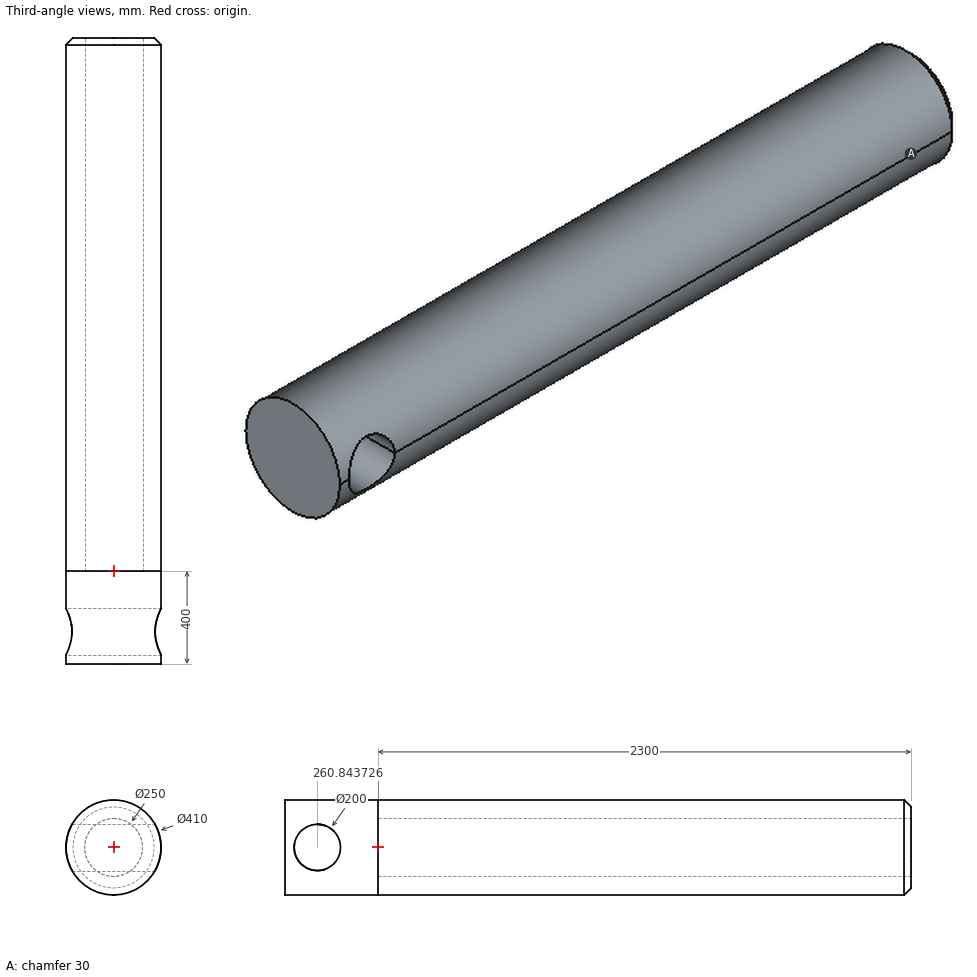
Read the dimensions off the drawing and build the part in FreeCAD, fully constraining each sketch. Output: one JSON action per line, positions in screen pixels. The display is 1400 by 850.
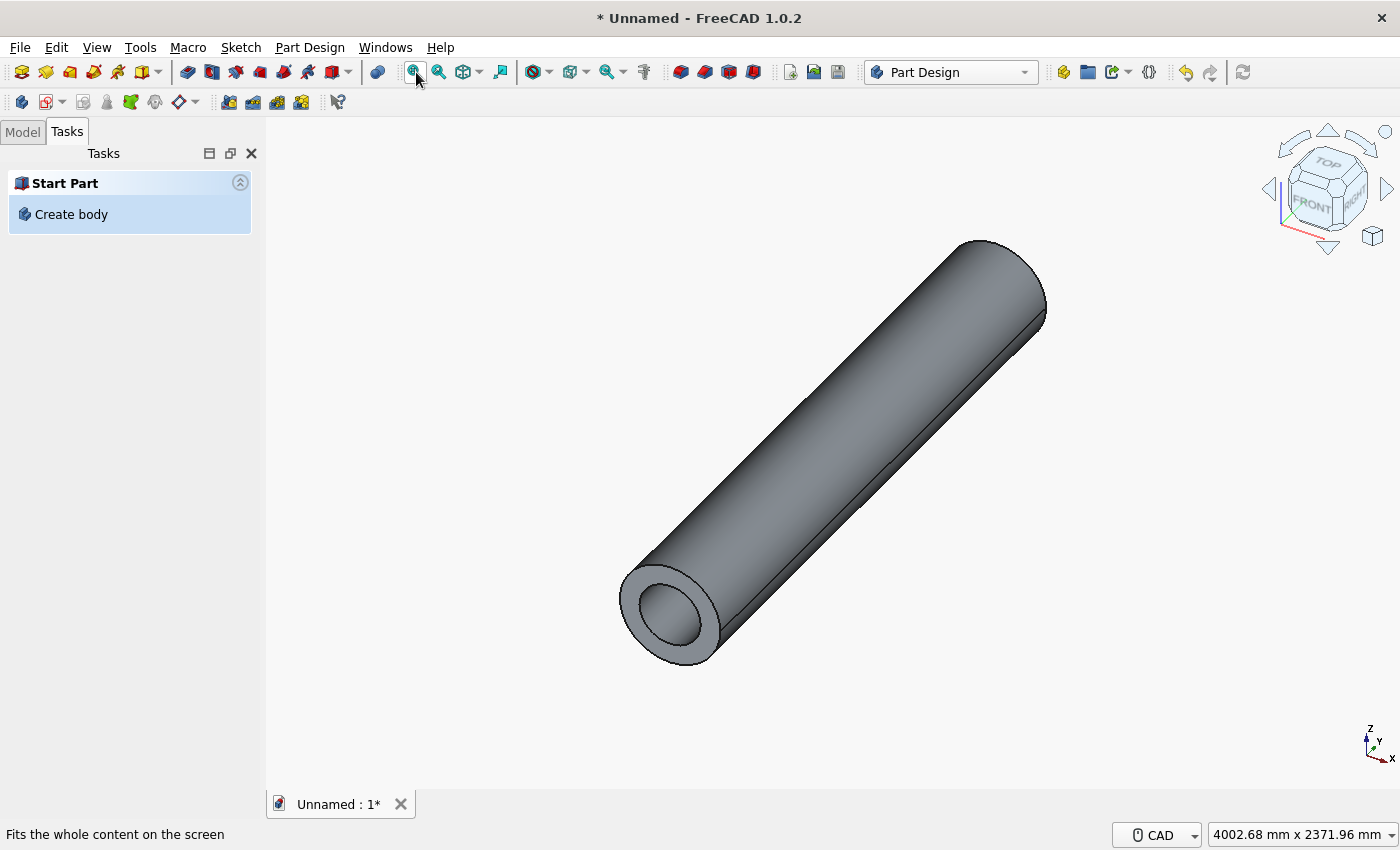
{"action": "left_click", "coordinate": [23, 131]}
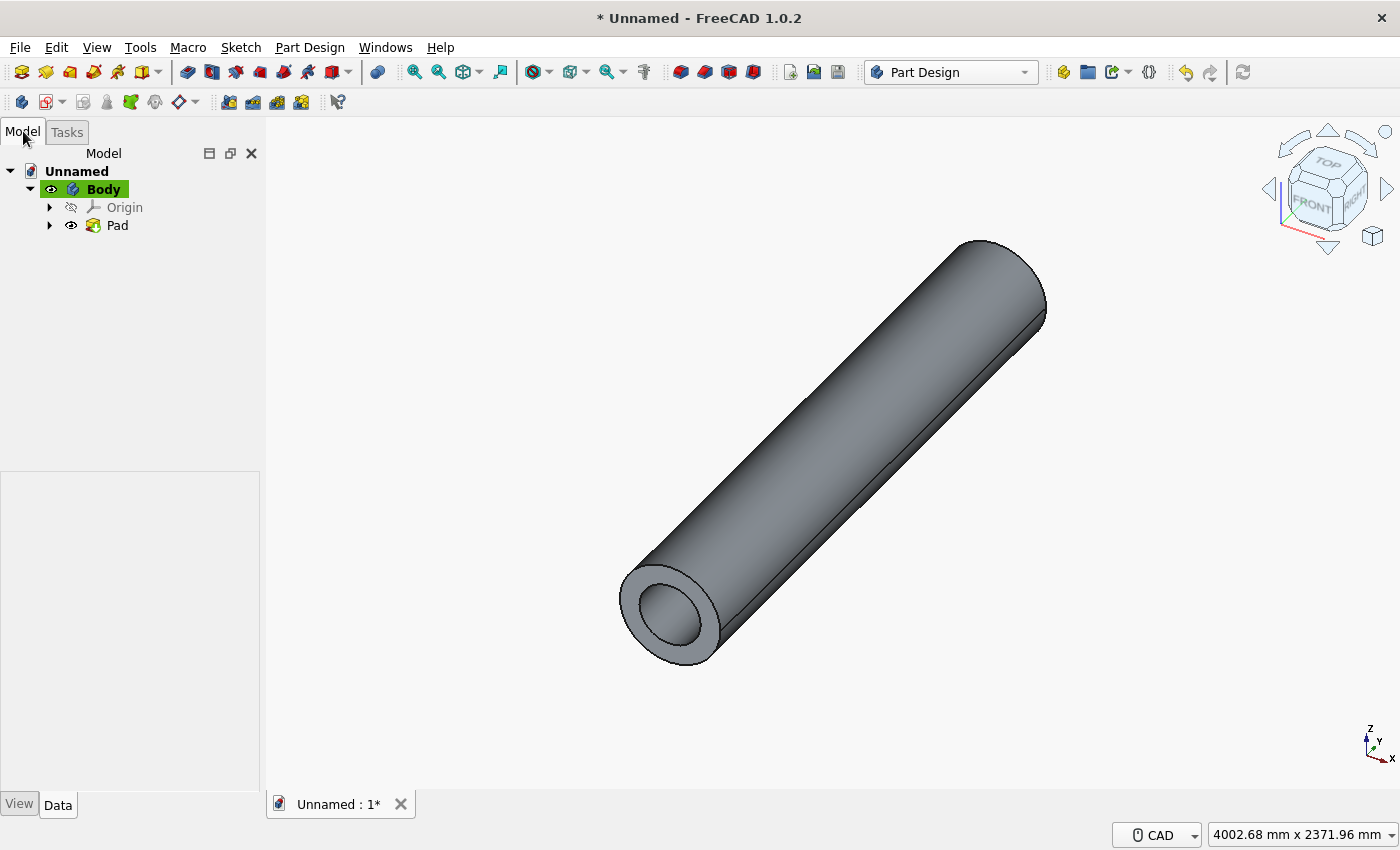
{"action": "left_click", "coordinate": [50, 207]}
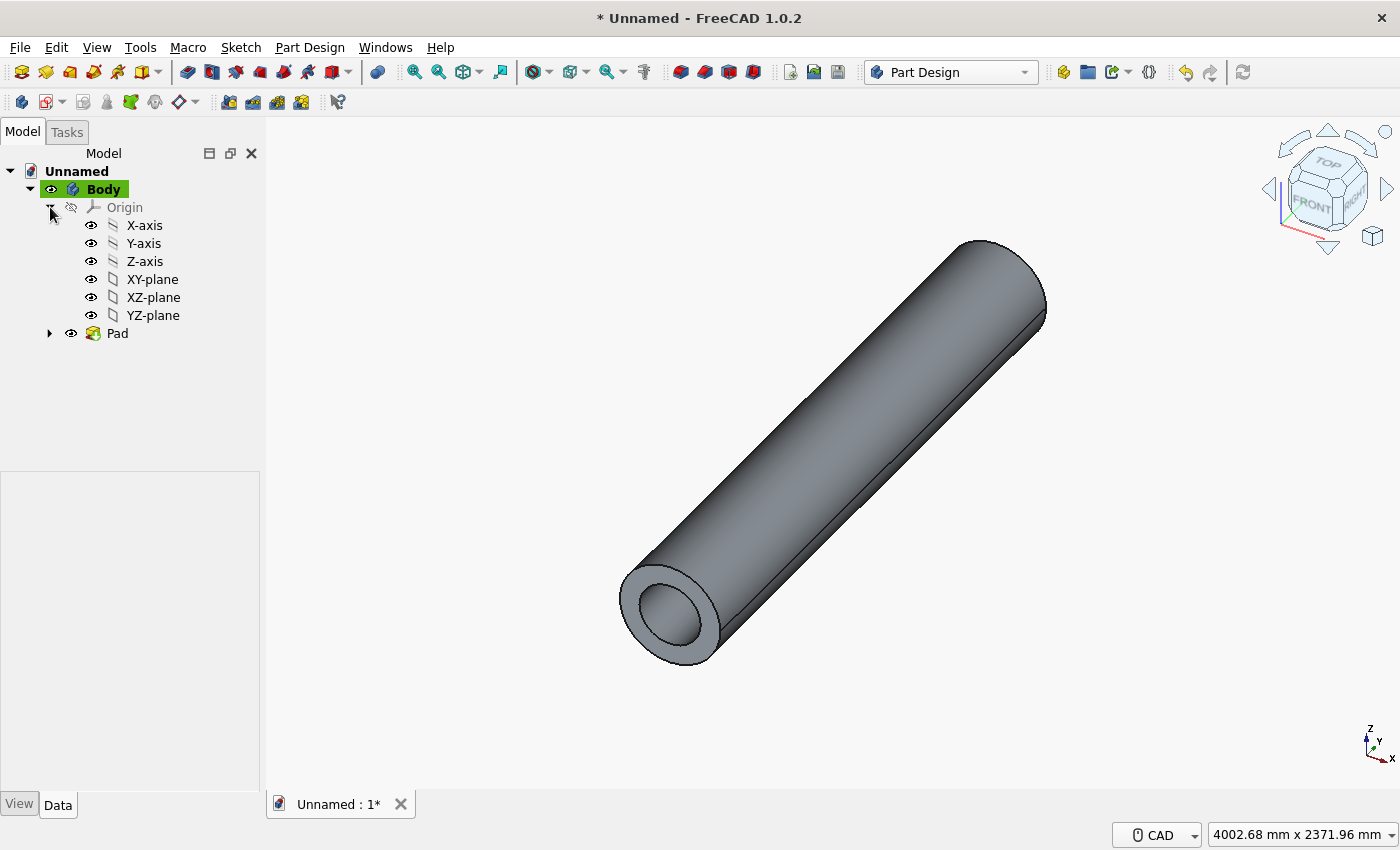
{"action": "left_click", "coordinate": [136, 297]}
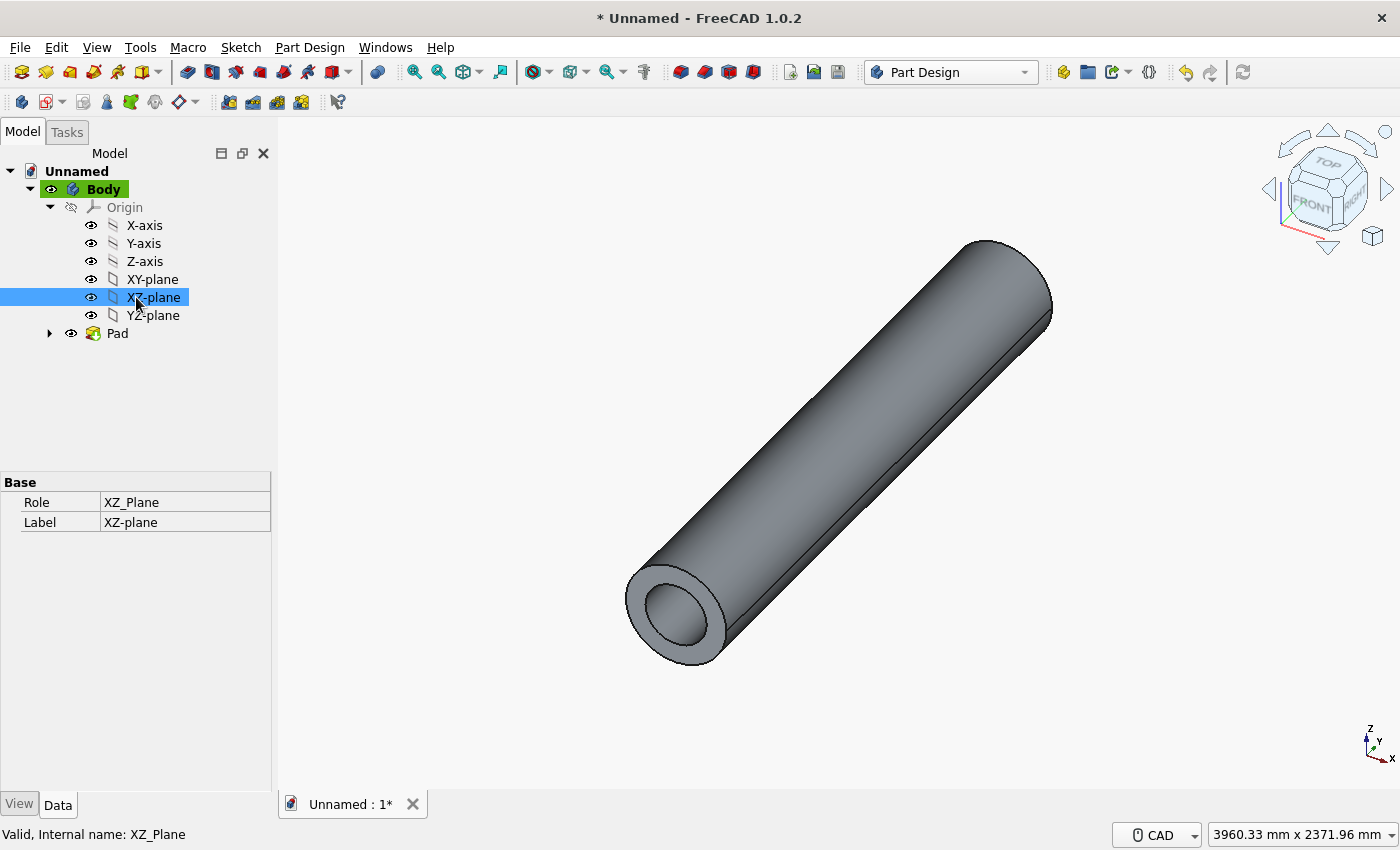
{"action": "left_click", "coordinate": [180, 102]}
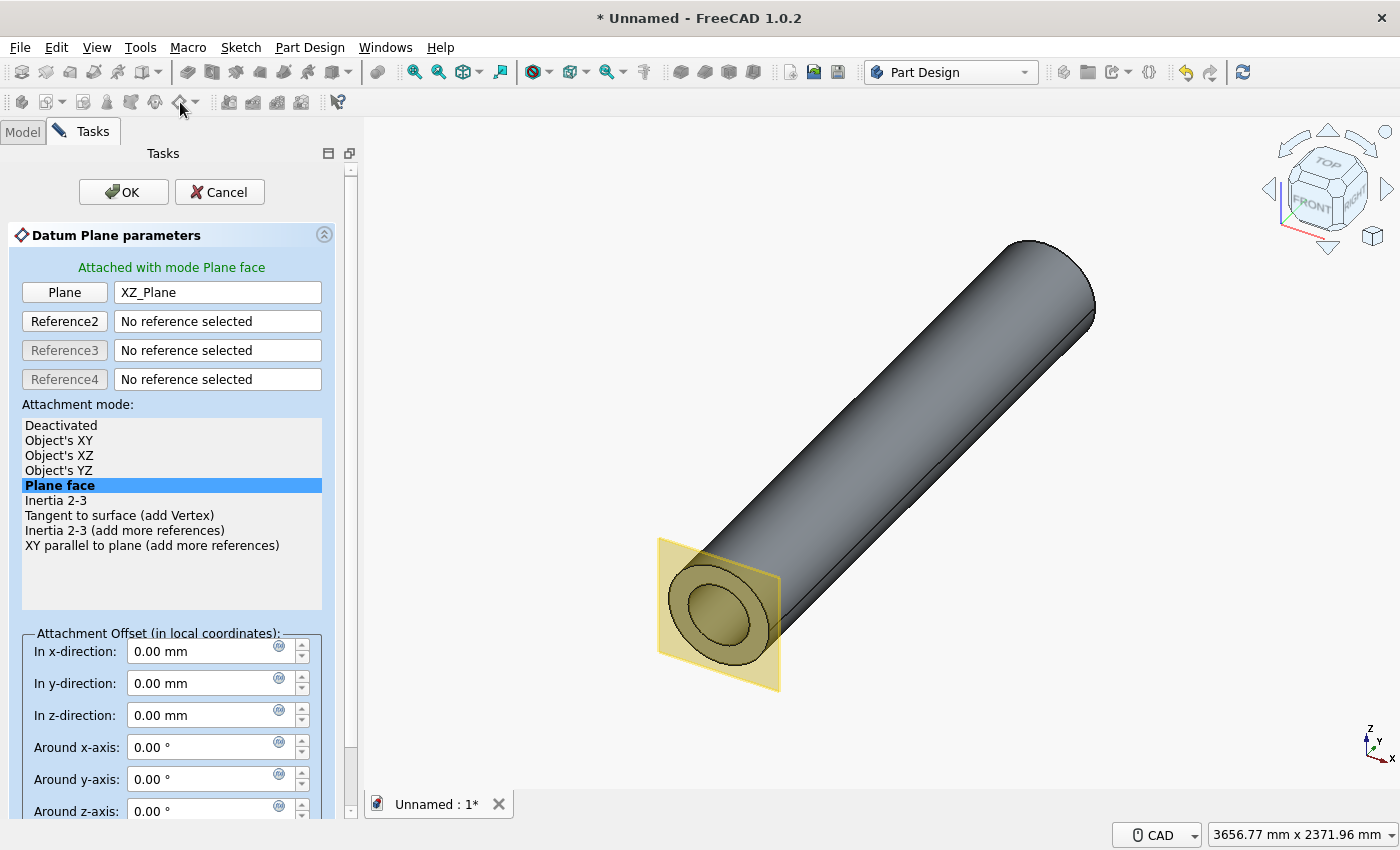
{"action": "triple_click", "coordinate": [210, 715]}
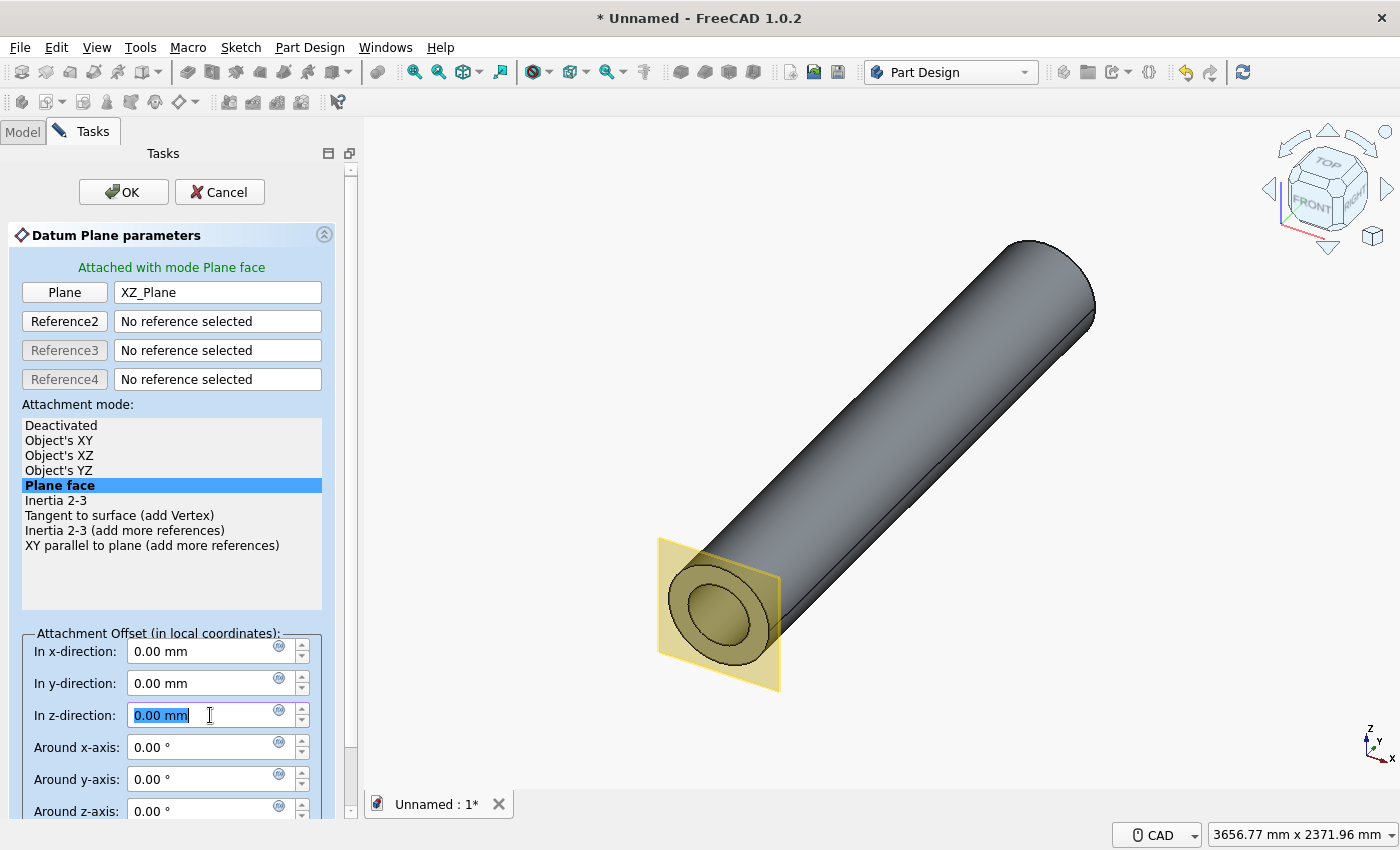
{"action": "type", "text": "400"}
{"action": "key", "text": "Tab"}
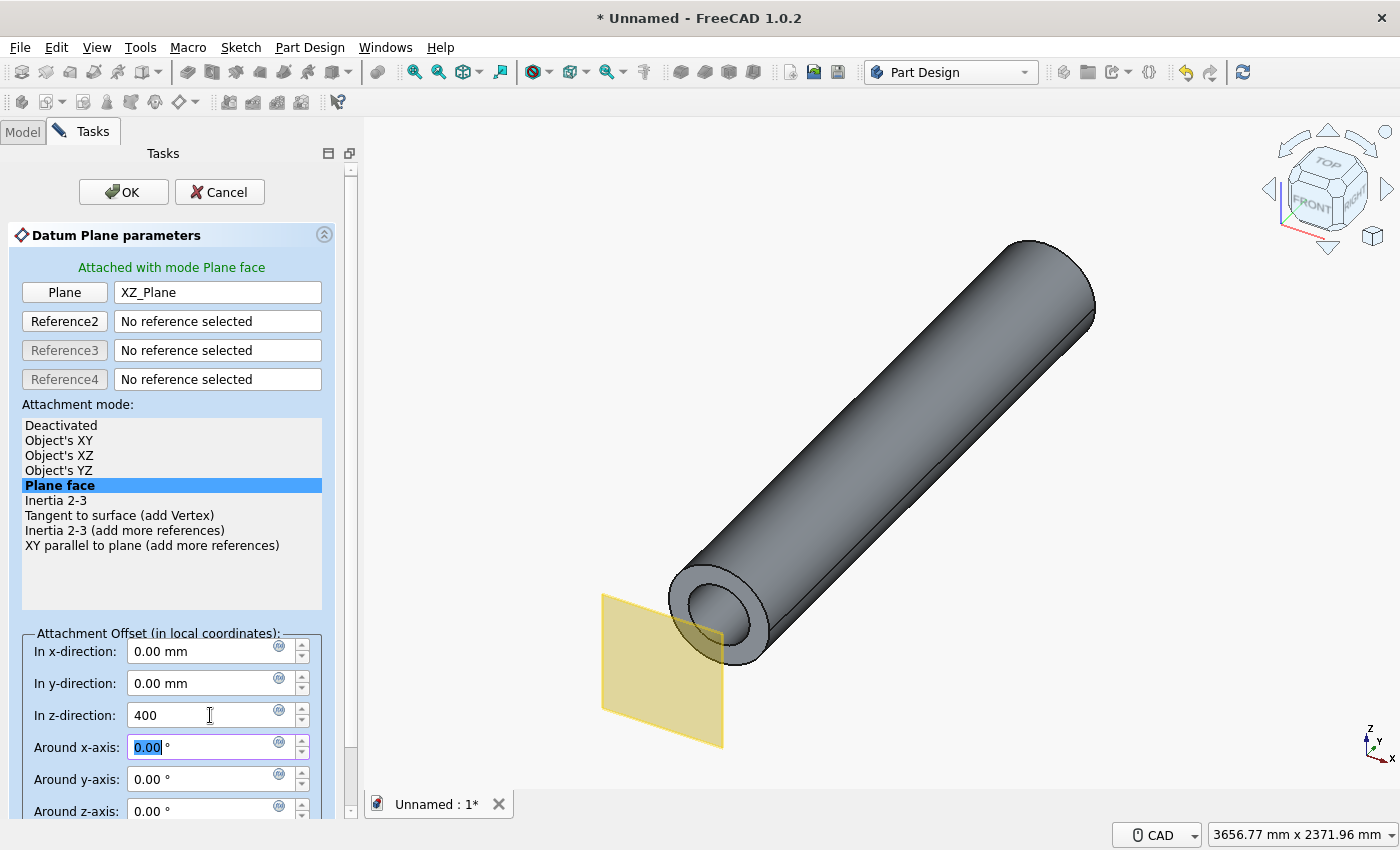
{"action": "left_click", "coordinate": [124, 192]}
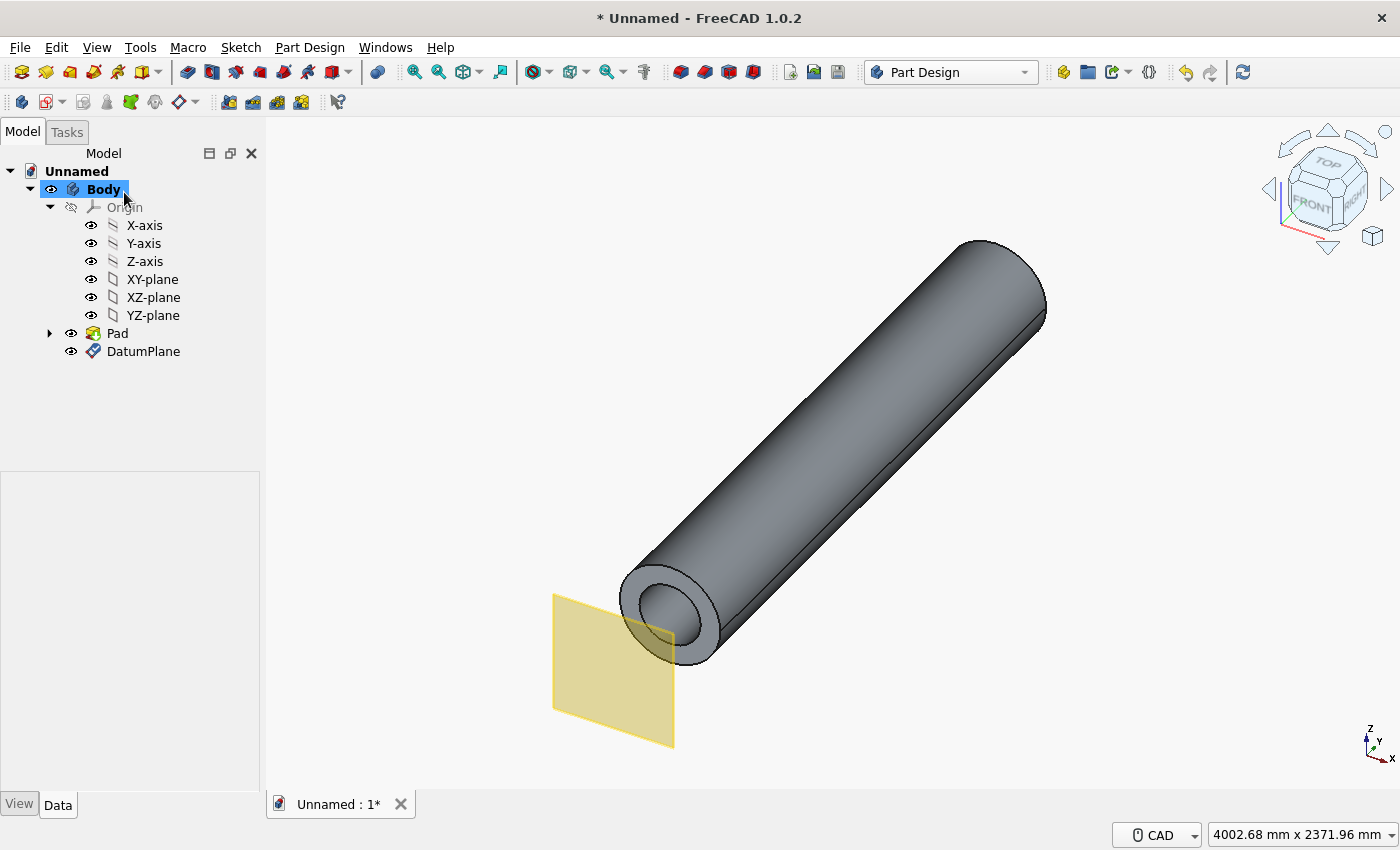
{"action": "left_click", "coordinate": [116, 351]}